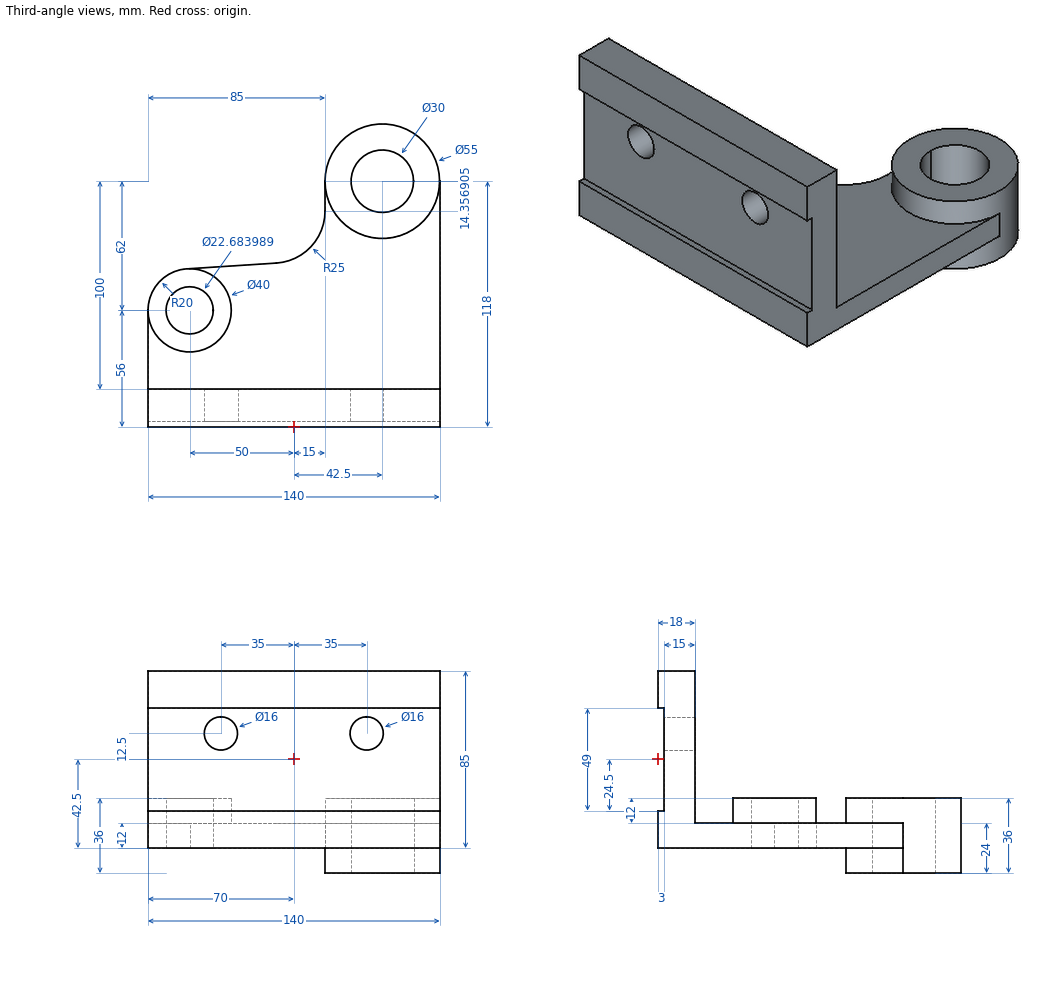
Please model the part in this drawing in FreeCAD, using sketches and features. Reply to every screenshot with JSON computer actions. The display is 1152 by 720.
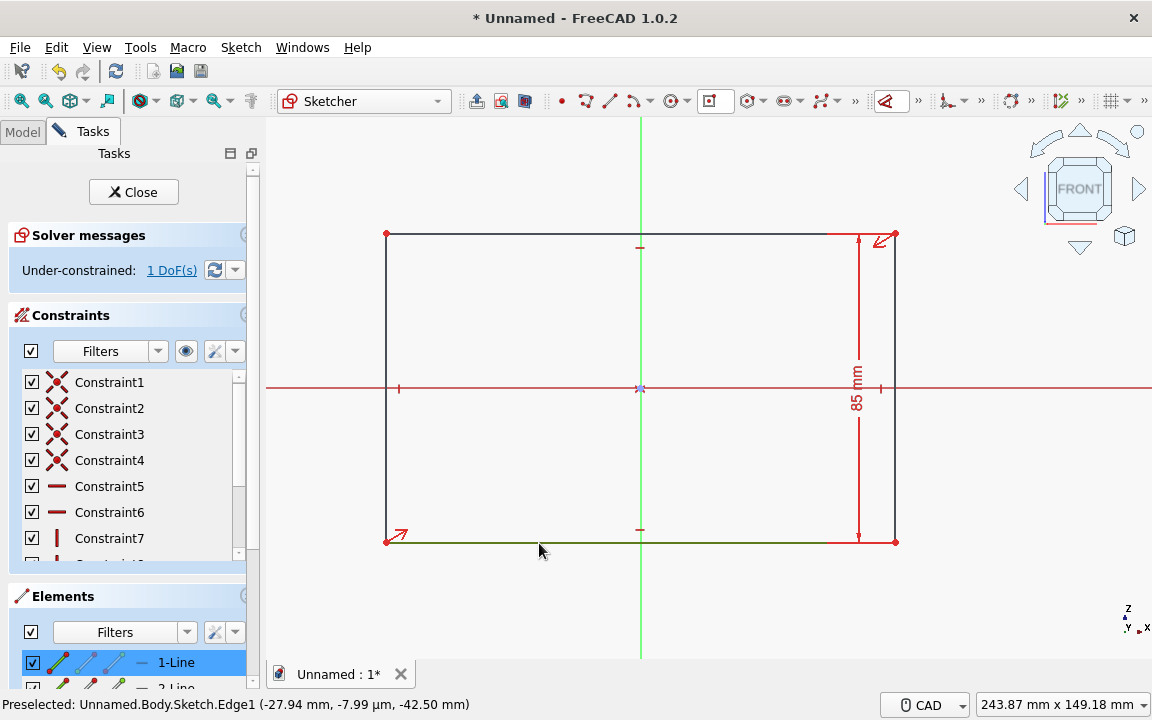
{"action": "key", "text": "l"}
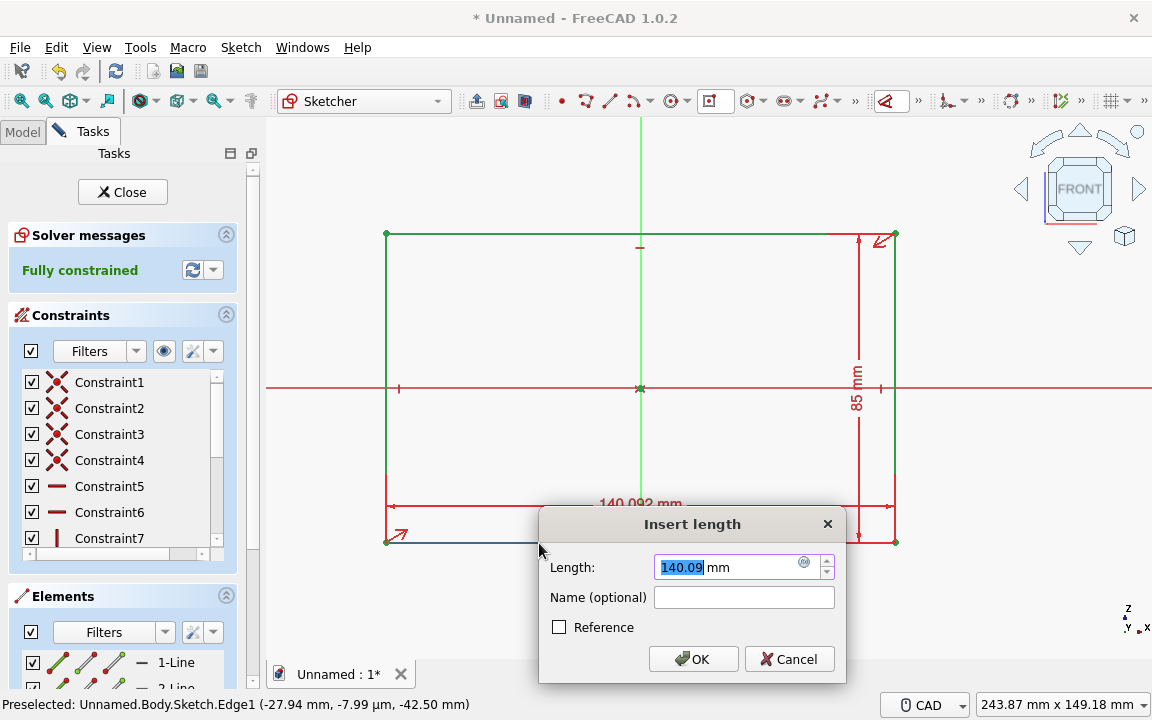
{"action": "type", "text": "140"}
{"action": "key", "text": "Return"}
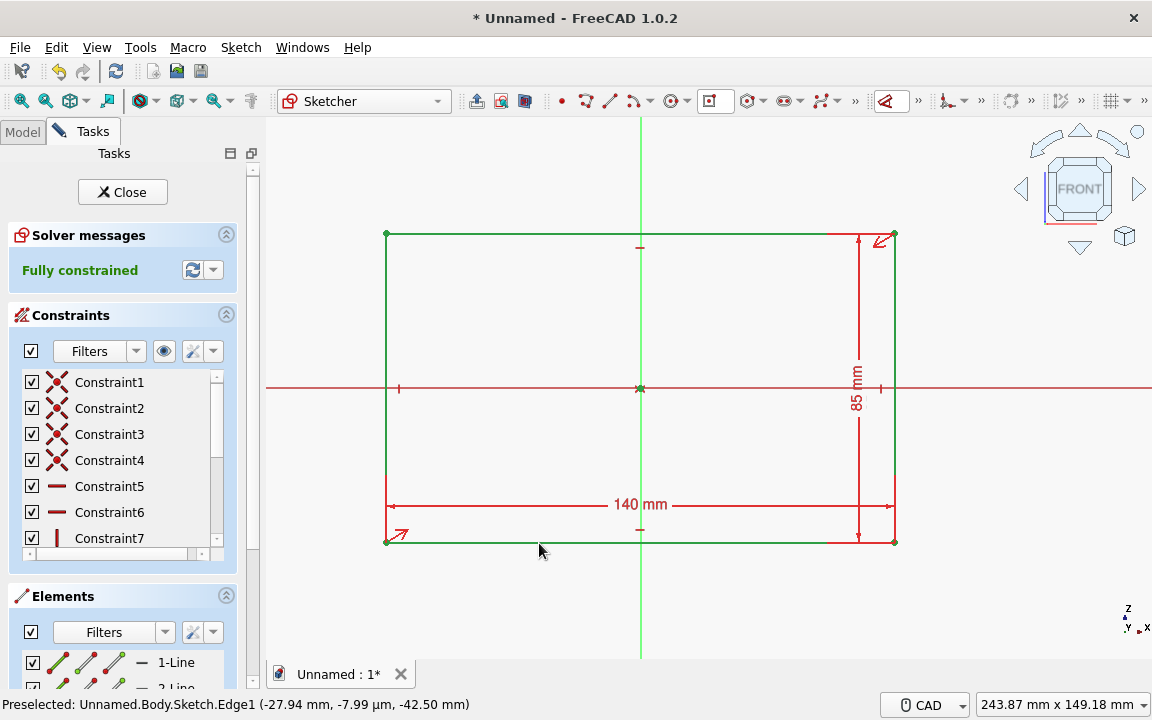
{"action": "left_click", "coordinate": [123, 192]}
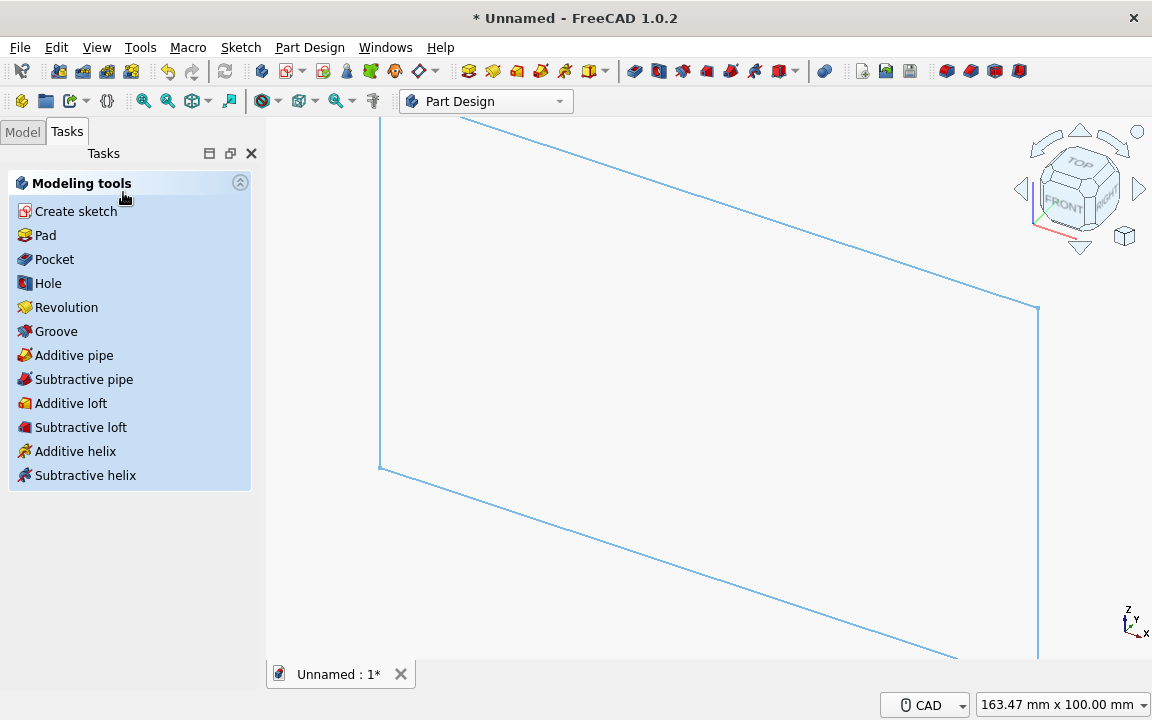
{"action": "left_click", "coordinate": [470, 72]}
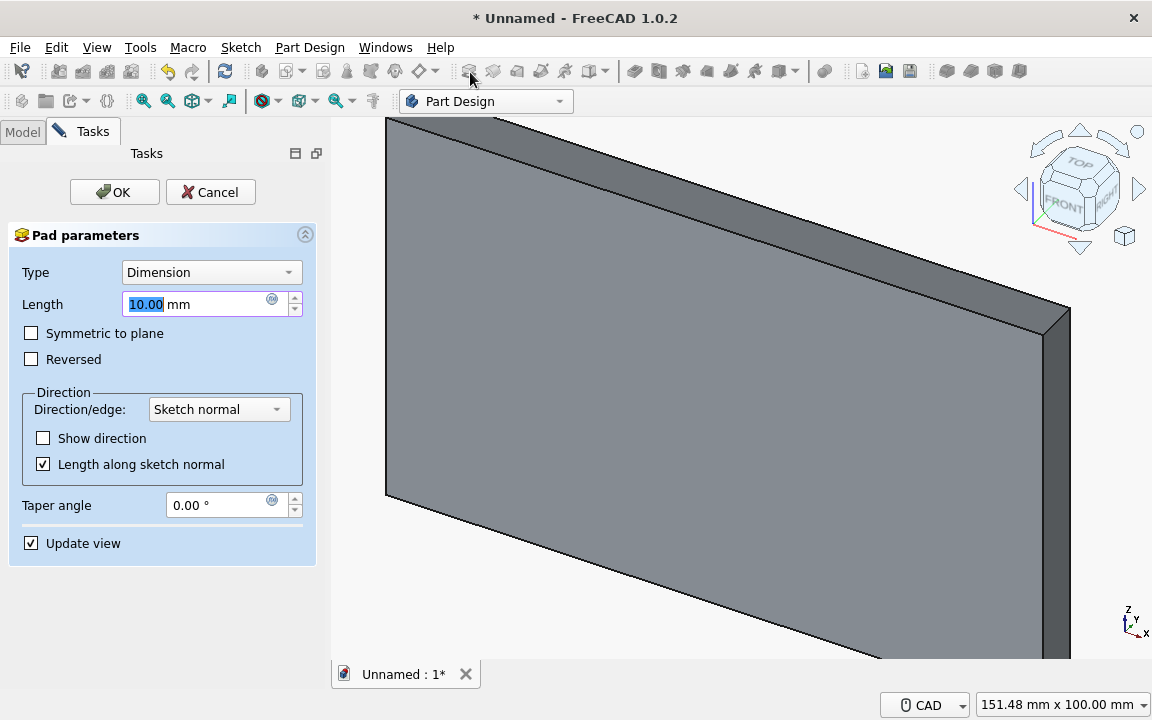
{"action": "type", "text": "18"}
{"action": "key", "text": "Tab"}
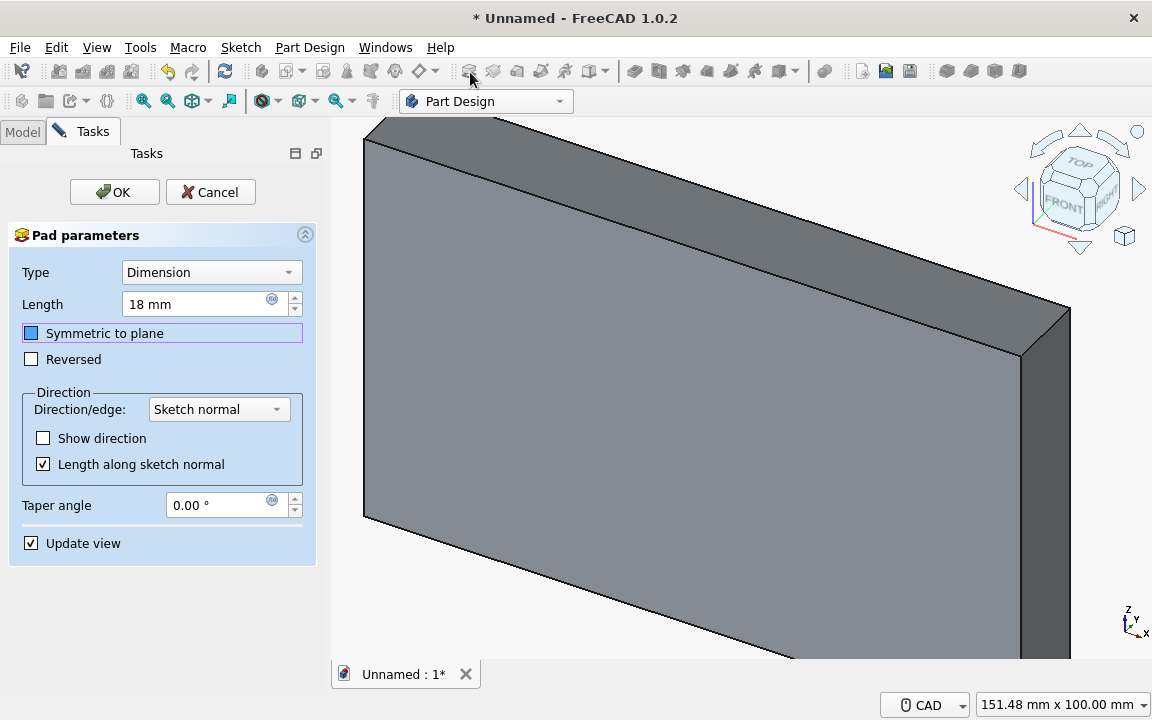
{"action": "left_click", "coordinate": [30, 359]}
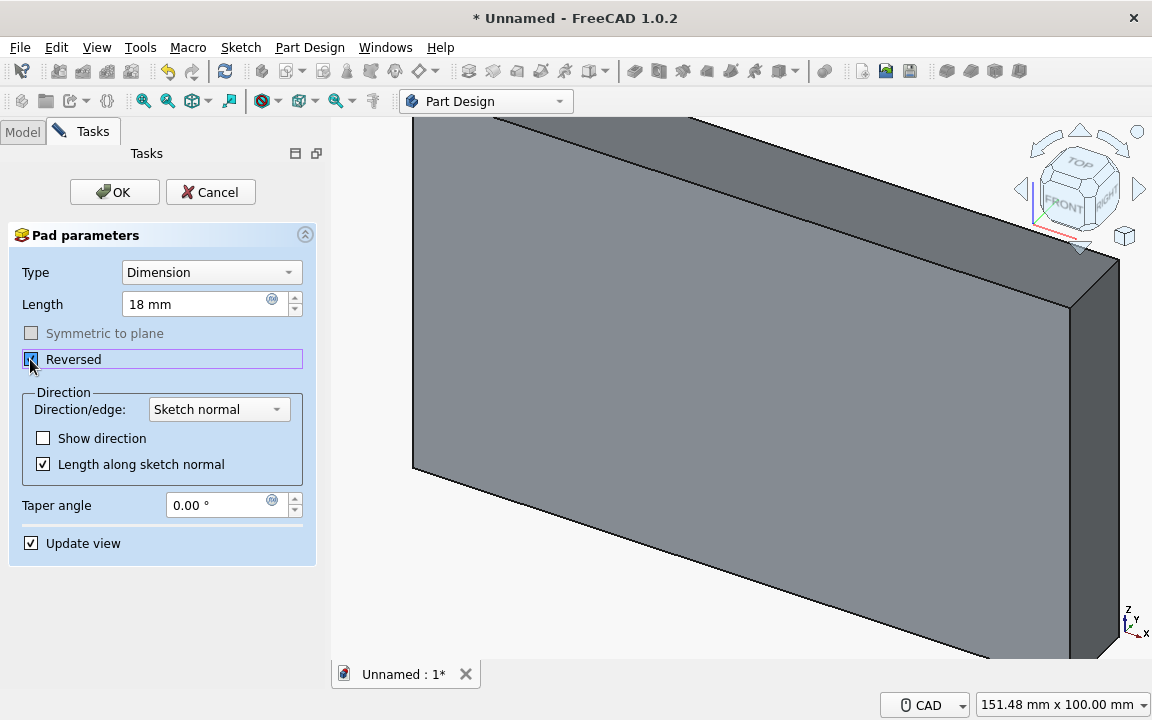
{"action": "left_click", "coordinate": [115, 192]}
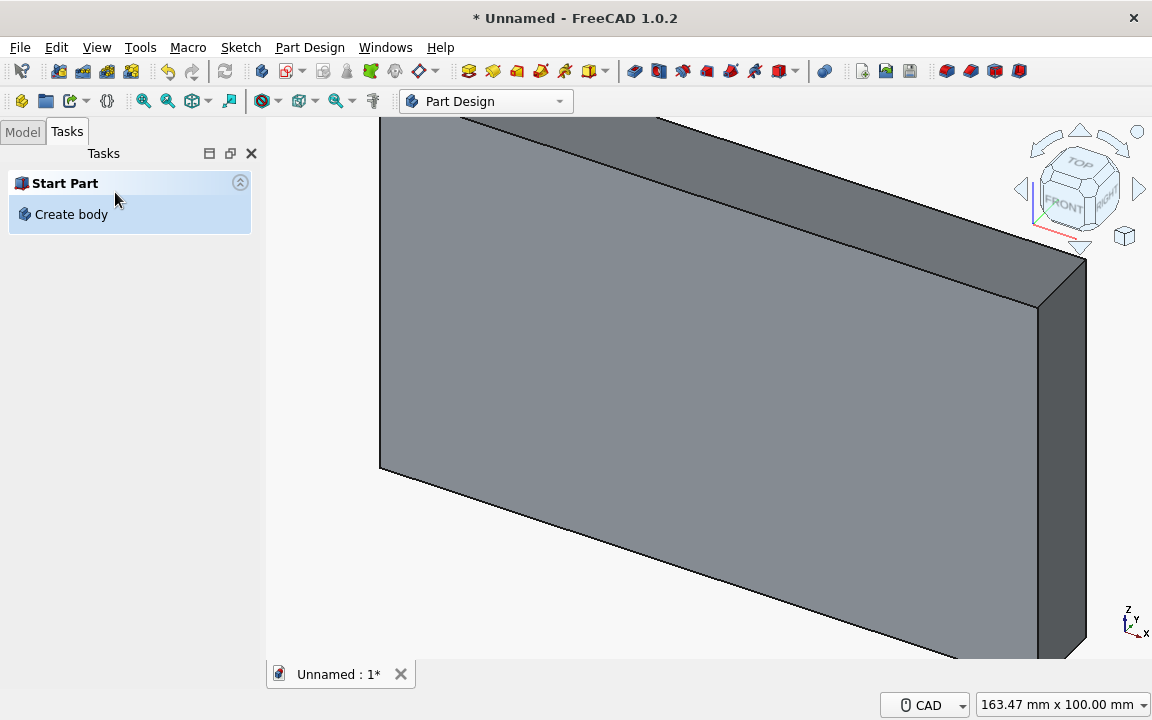
{"action": "key", "text": "v f"}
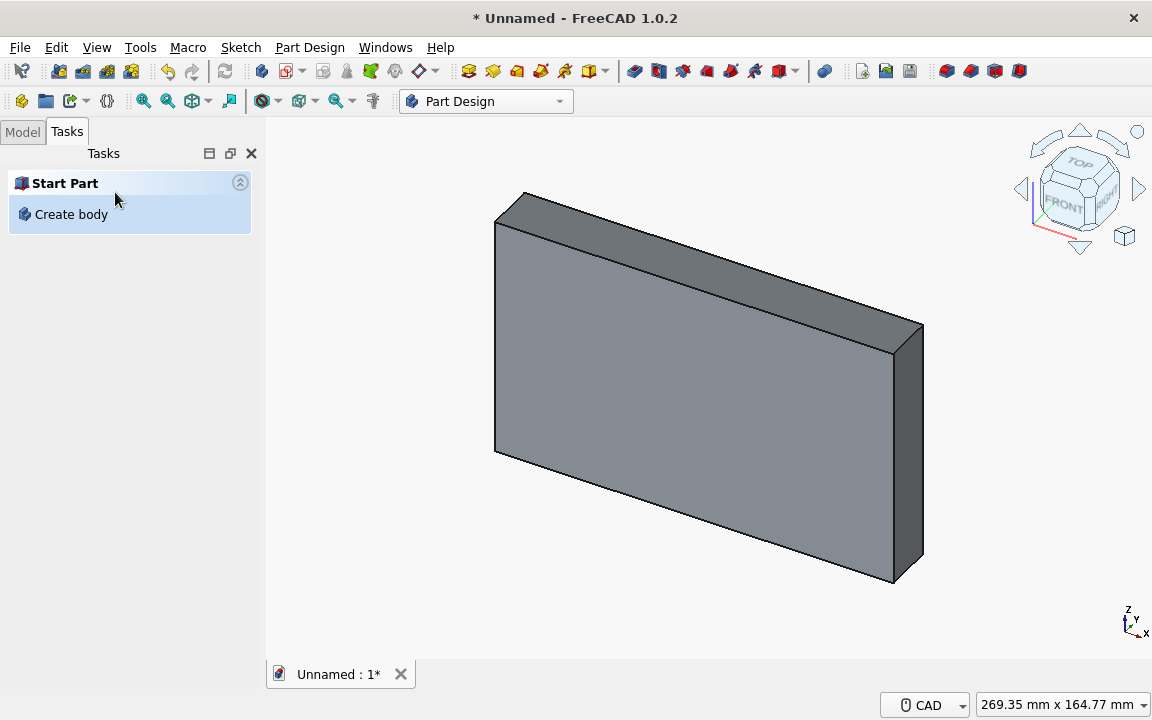
{"action": "left_click", "coordinate": [908, 453]}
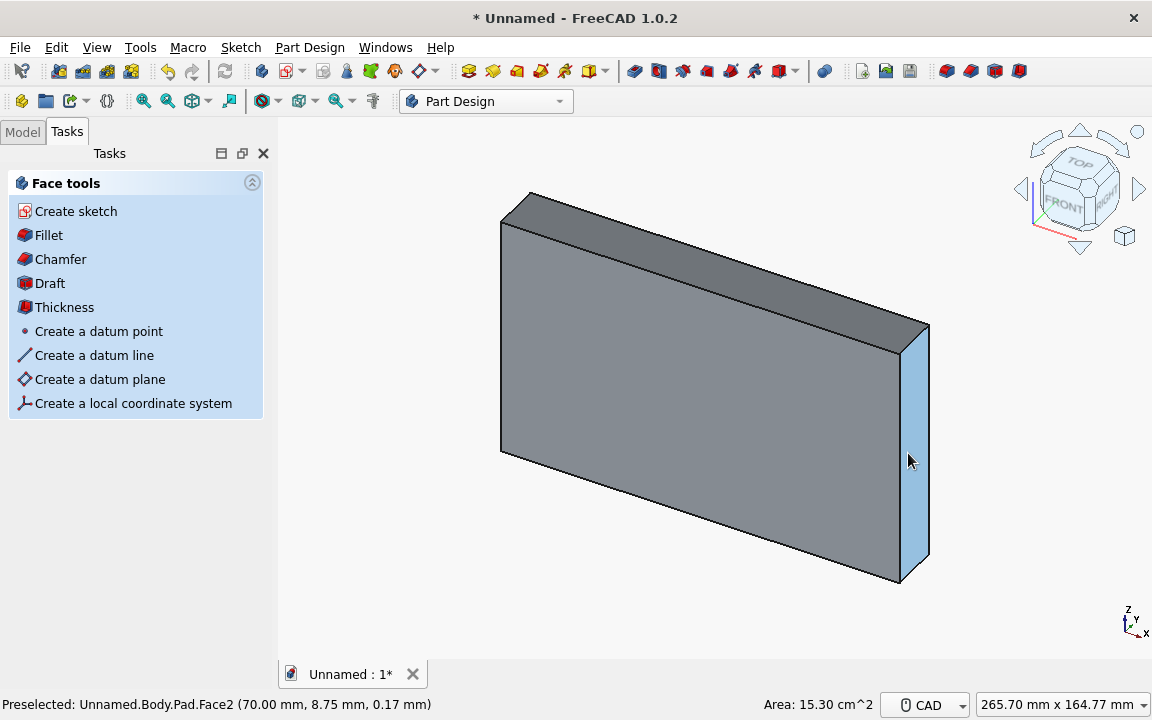
{"action": "left_click", "coordinate": [286, 72]}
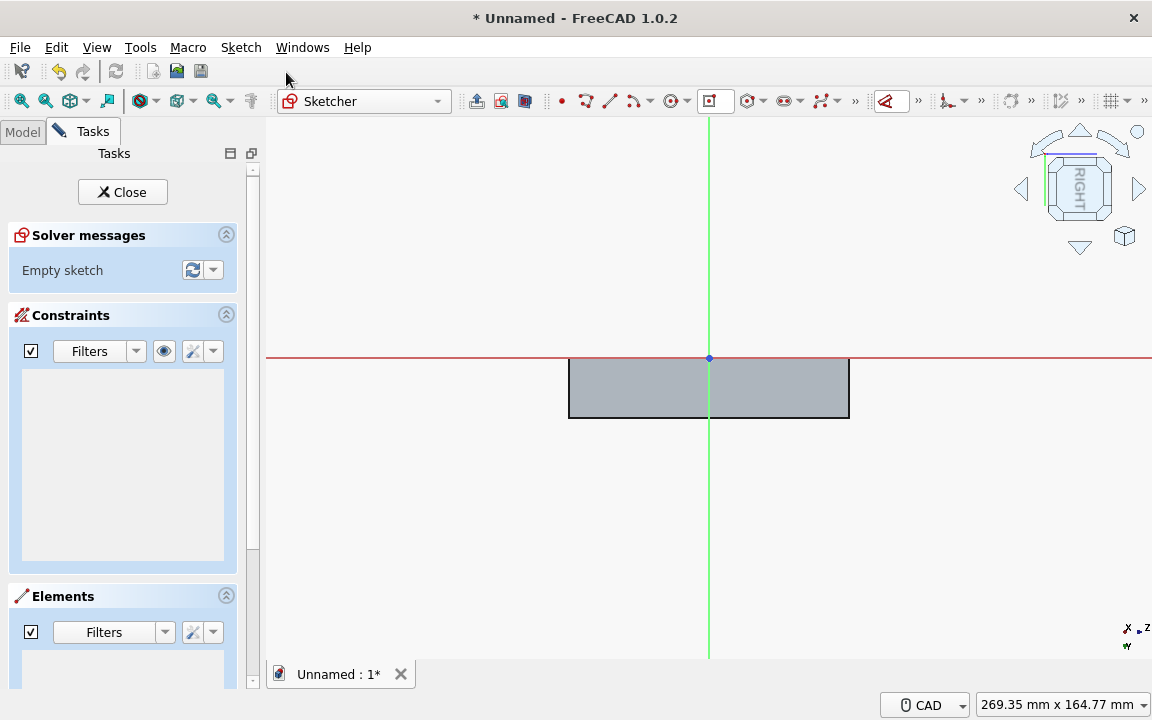
{"action": "scroll", "coordinate": [739, 353], "scroll_direction": "up", "scroll_amount": 6}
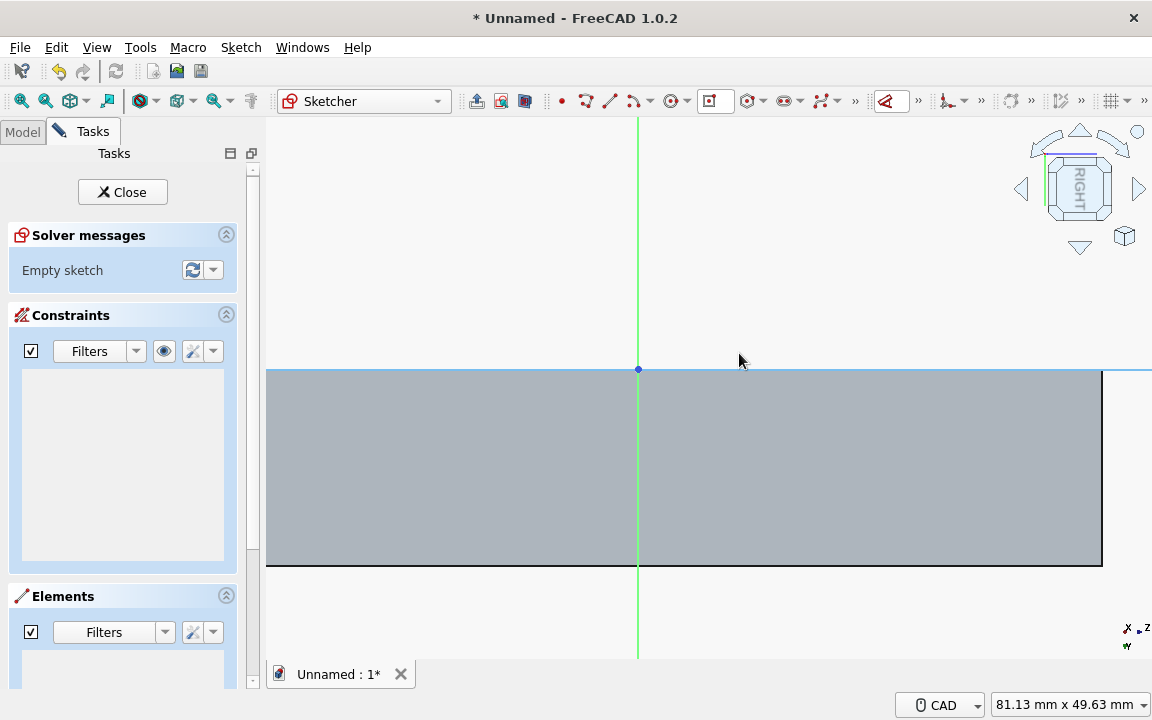
{"action": "key", "text": "g r"}